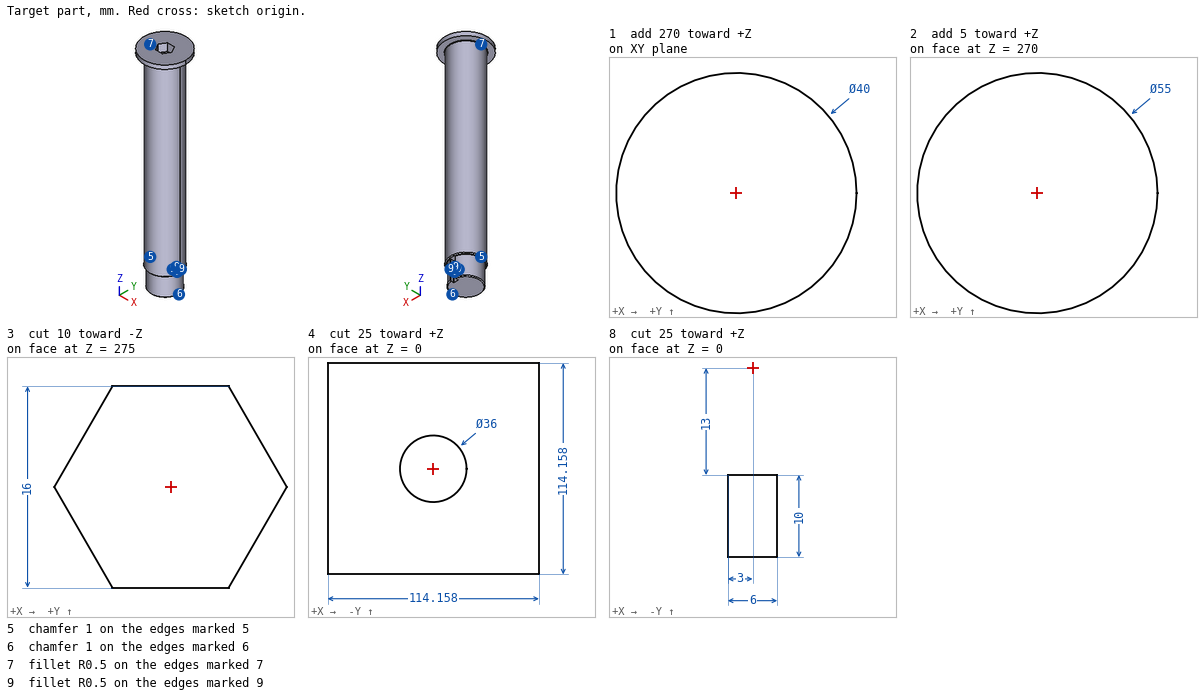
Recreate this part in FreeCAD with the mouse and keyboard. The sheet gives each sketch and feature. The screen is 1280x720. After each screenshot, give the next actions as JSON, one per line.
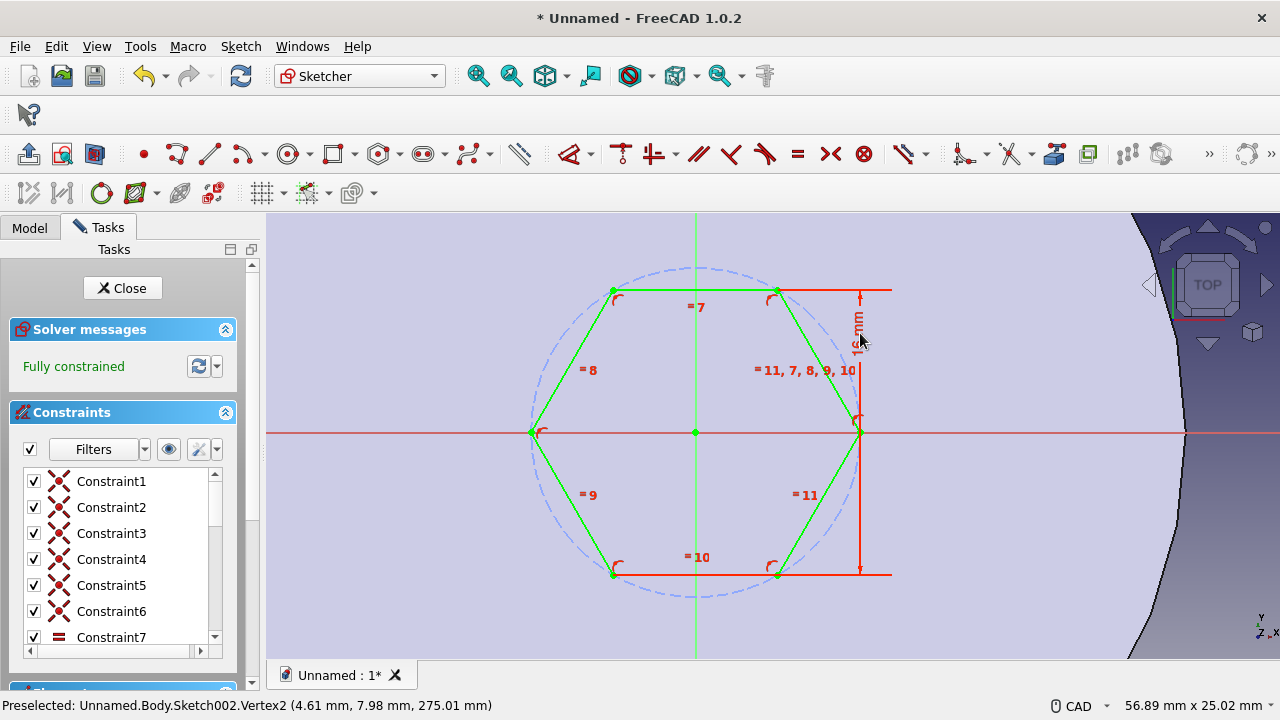
{"action": "left_click", "coordinate": [123, 288]}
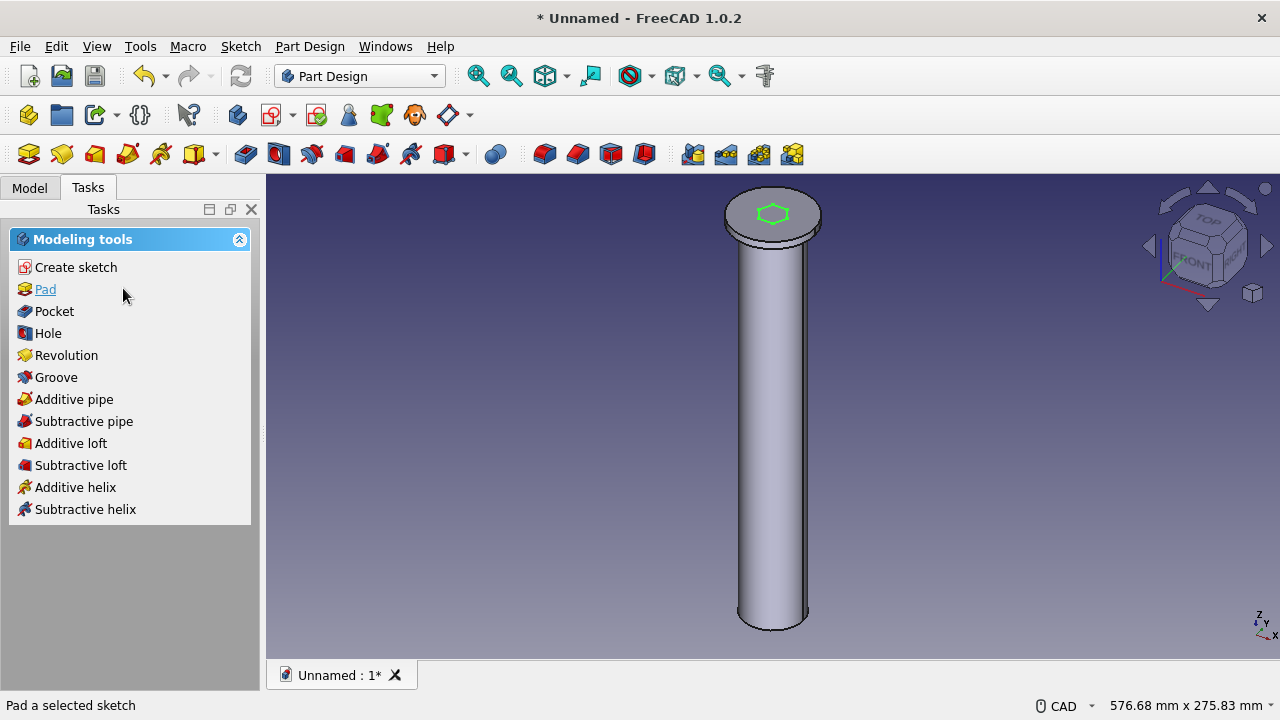
{"action": "left_click", "coordinate": [246, 154]}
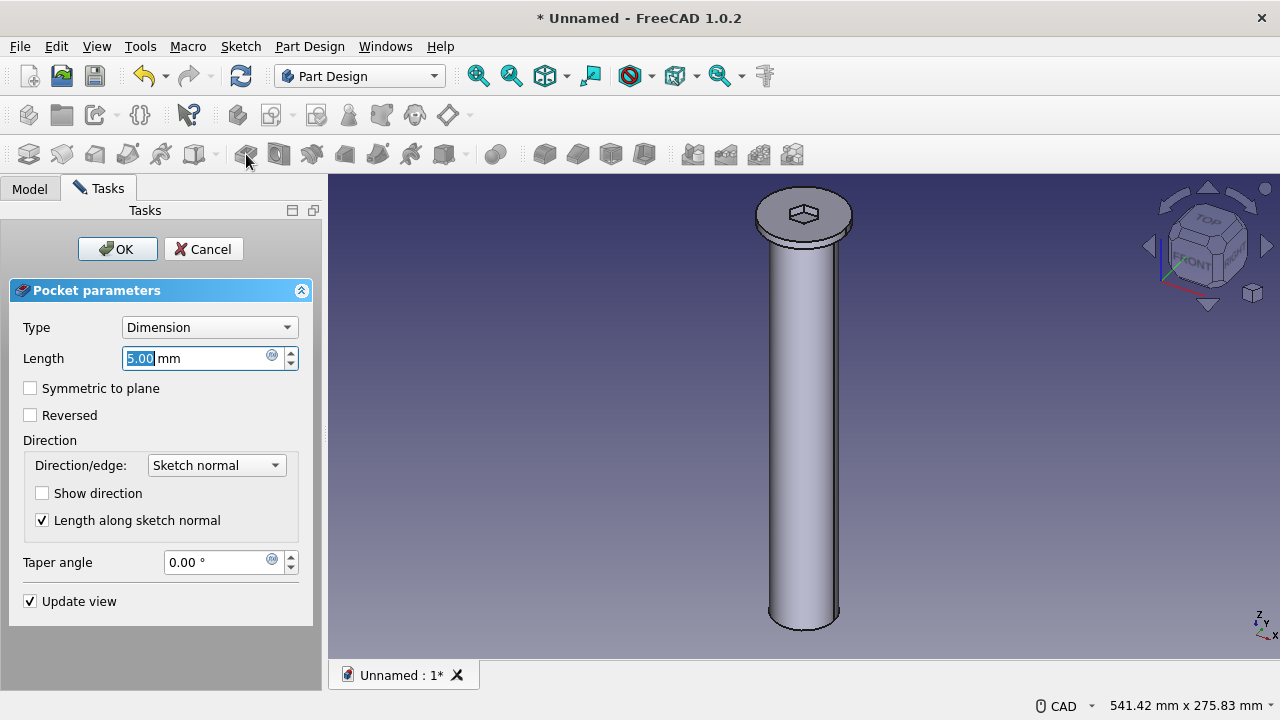
{"action": "type", "text": "10"}
{"action": "key", "text": "Tab"}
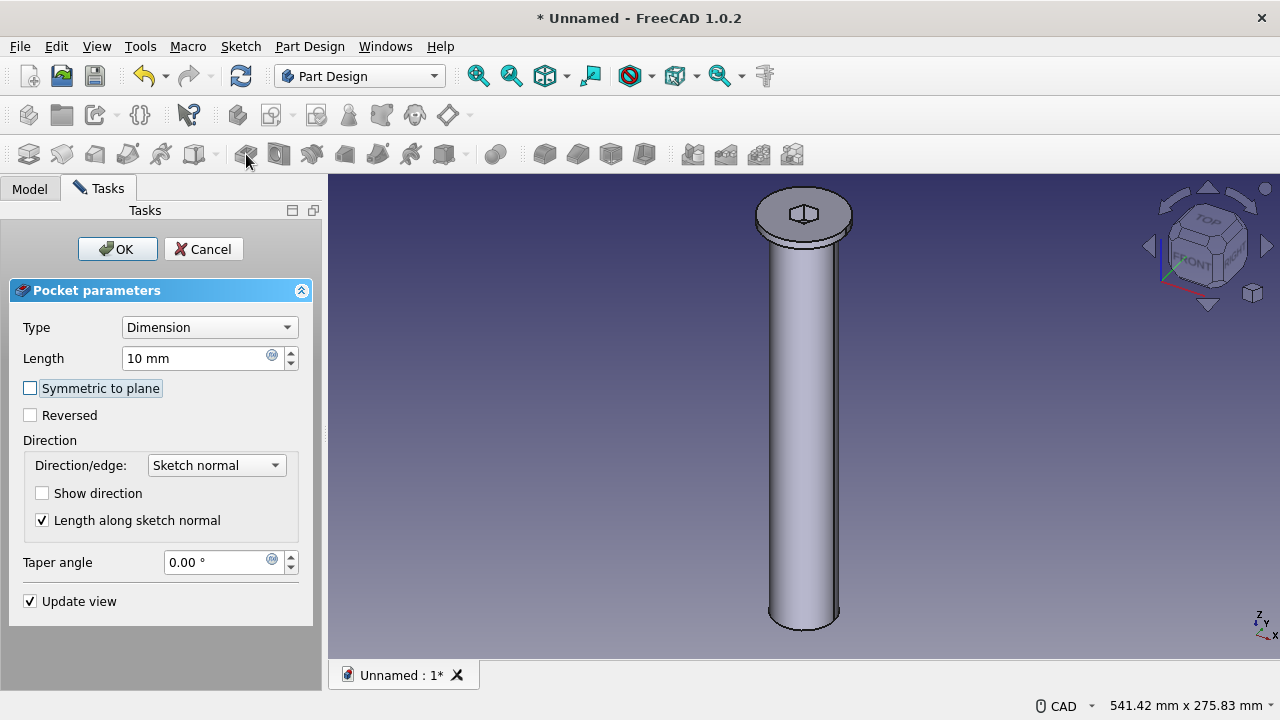
{"action": "left_click", "coordinate": [118, 249]}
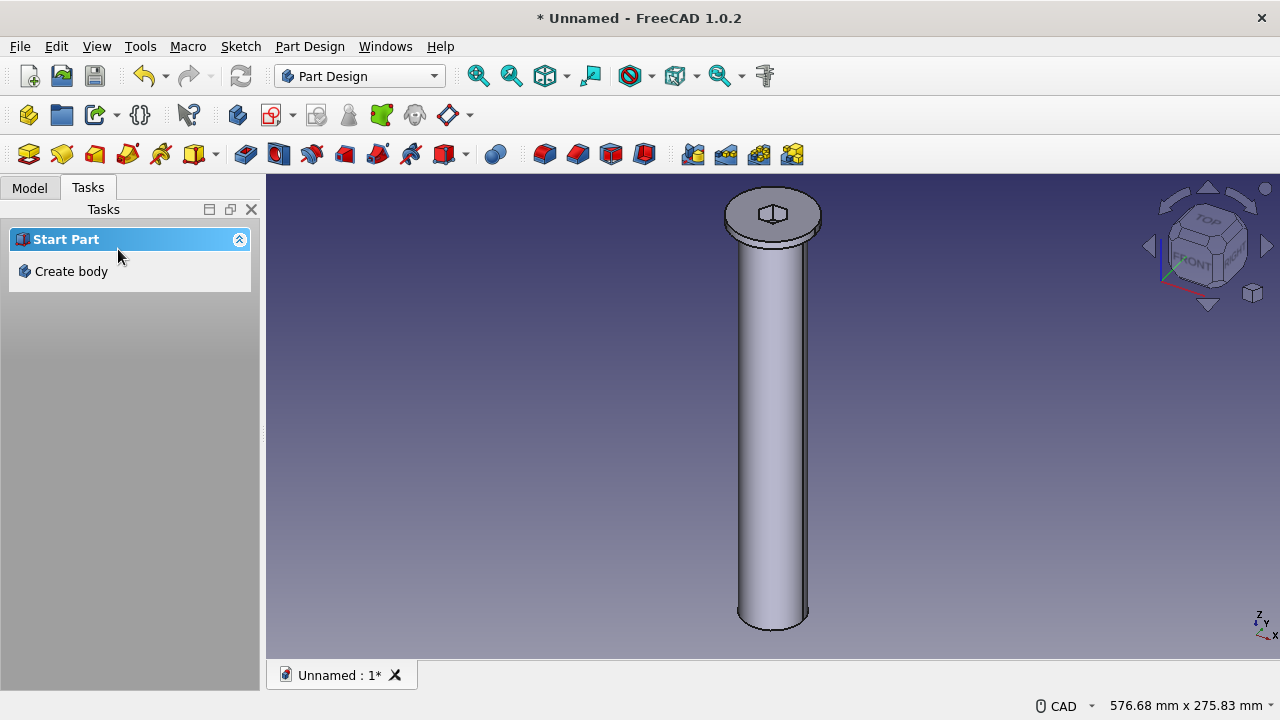
{"action": "key", "text": "5"}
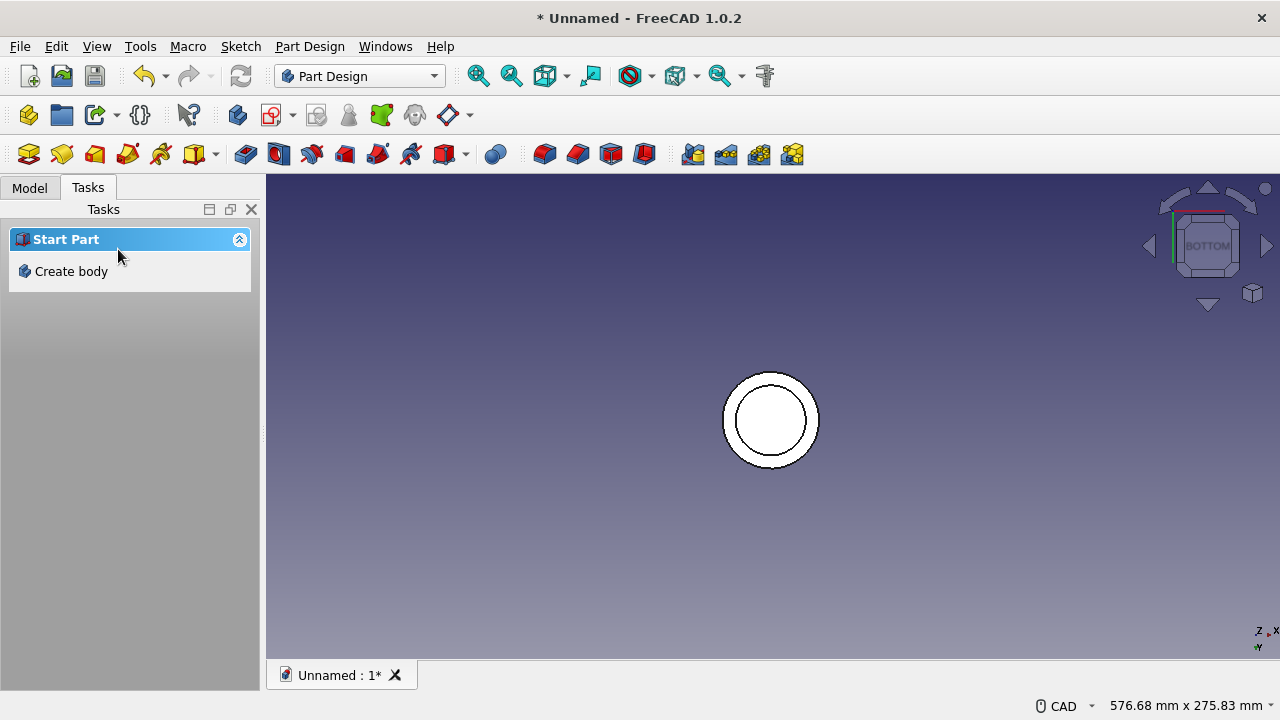
{"action": "left_click", "coordinate": [479, 76]}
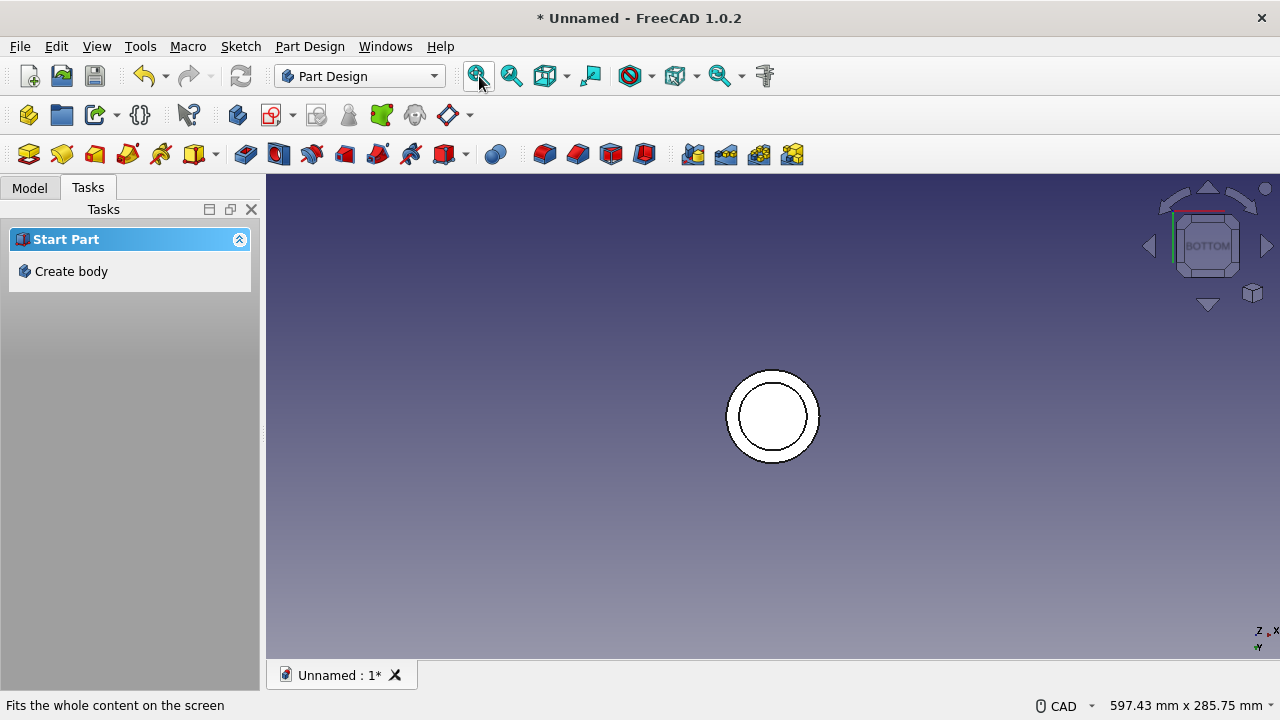
{"action": "left_click", "coordinate": [773, 415]}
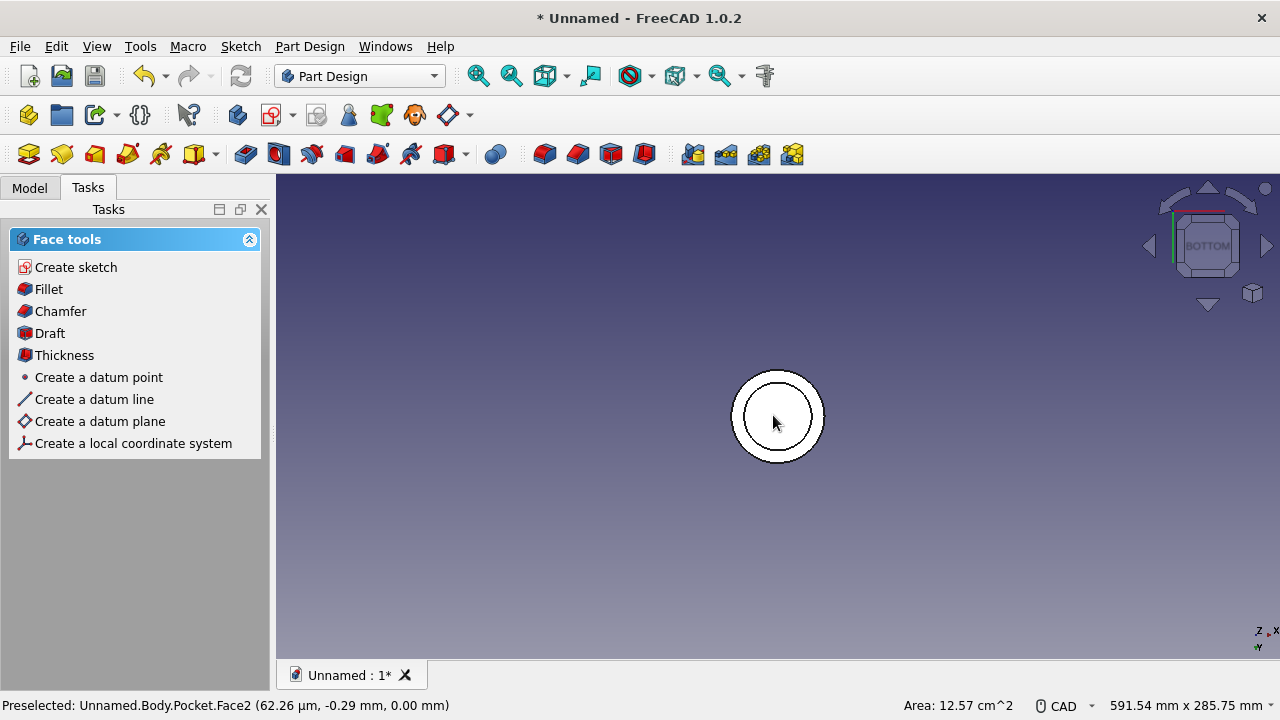
{"action": "left_click", "coordinate": [270, 116]}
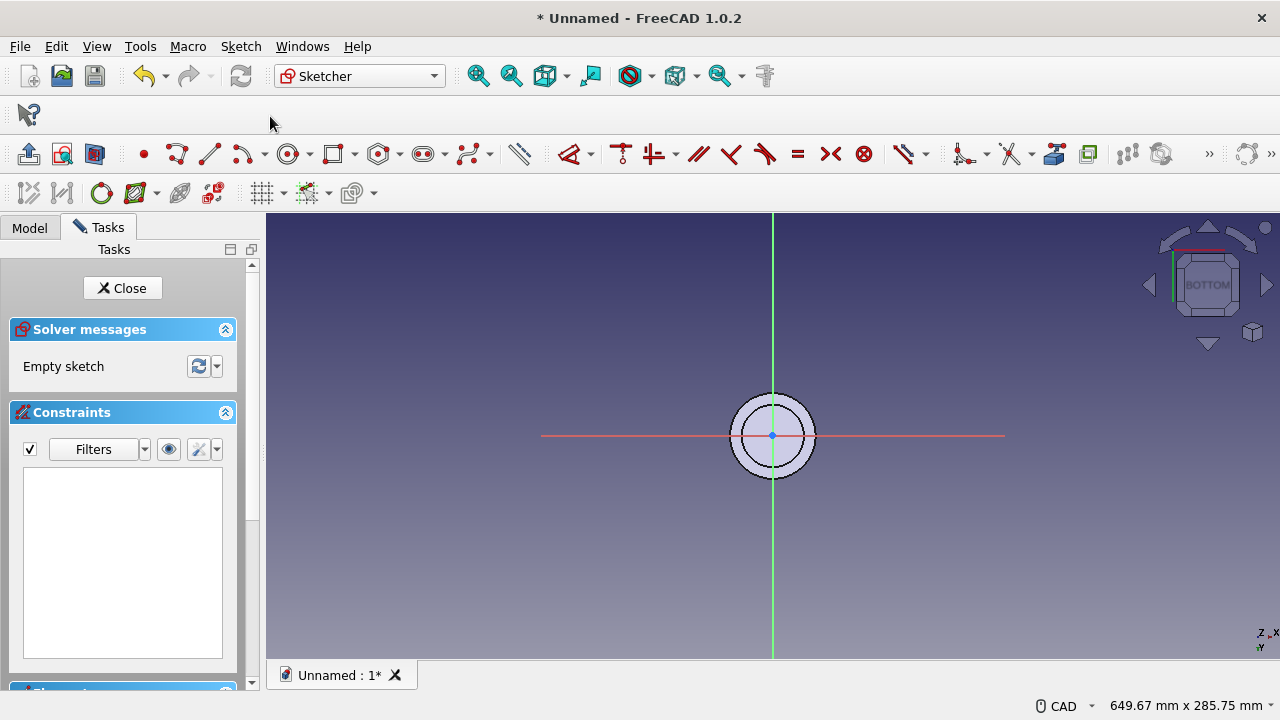
{"action": "scroll", "coordinate": [912, 436], "scroll_direction": "up", "scroll_amount": 2}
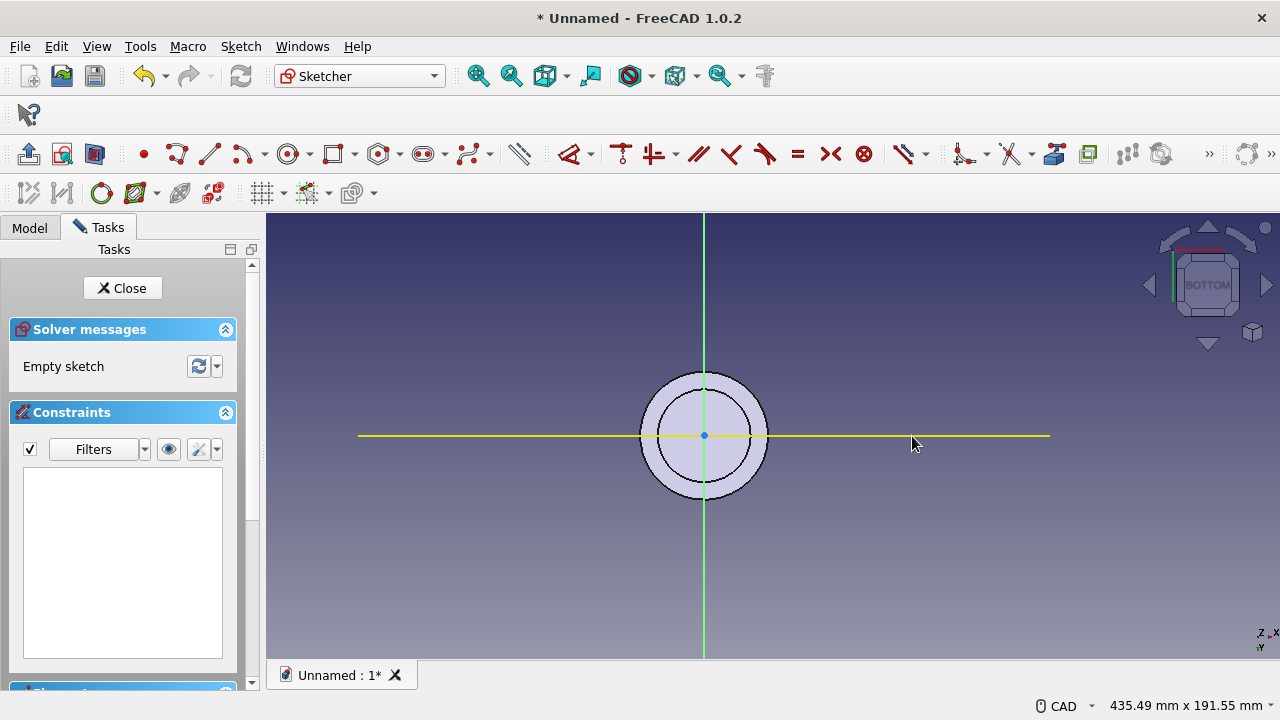
{"action": "key", "text": "g v"}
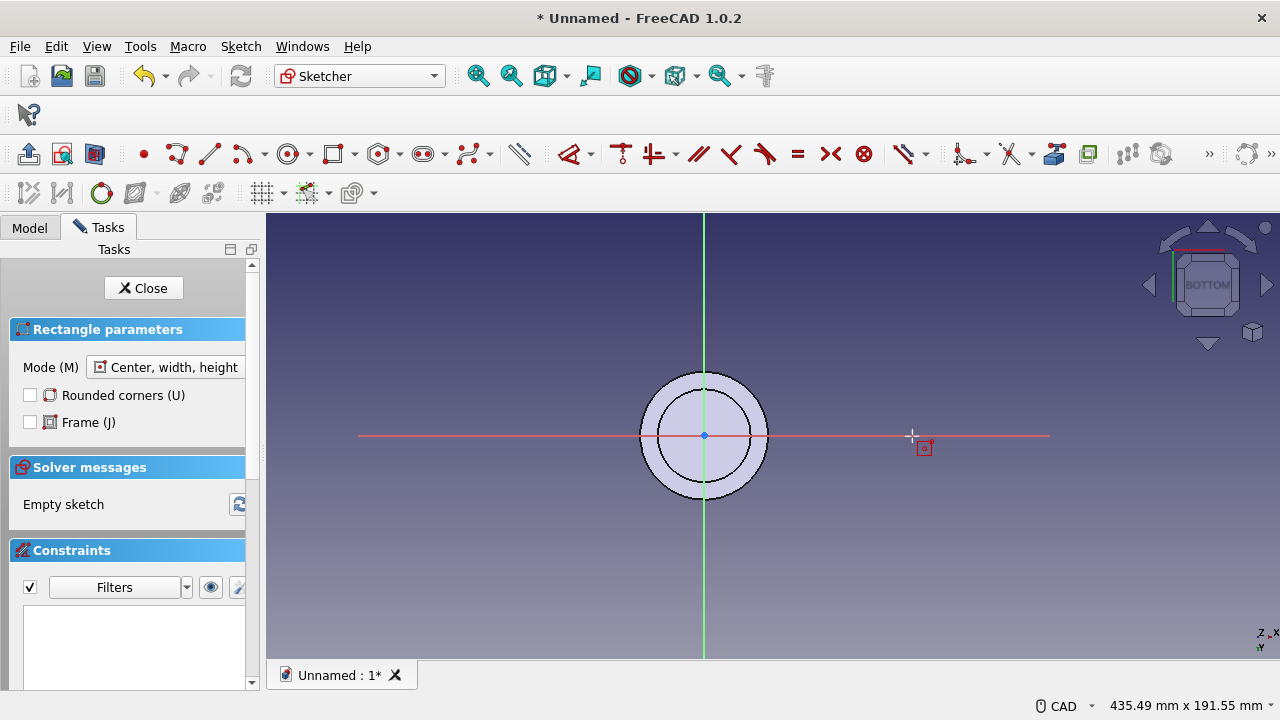
{"action": "left_click", "coordinate": [704, 436]}
{"action": "mouse_move", "coordinate": [837, 303]}